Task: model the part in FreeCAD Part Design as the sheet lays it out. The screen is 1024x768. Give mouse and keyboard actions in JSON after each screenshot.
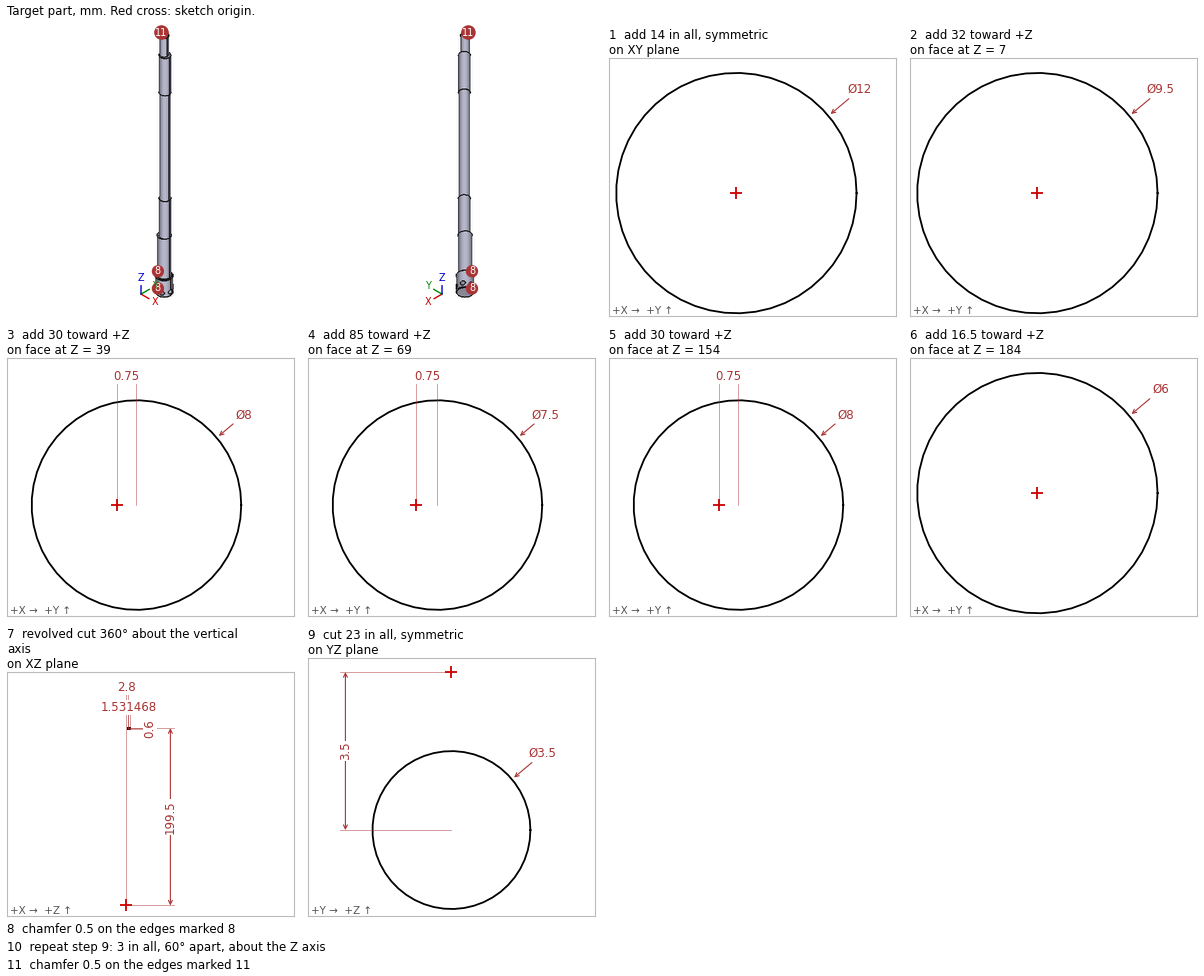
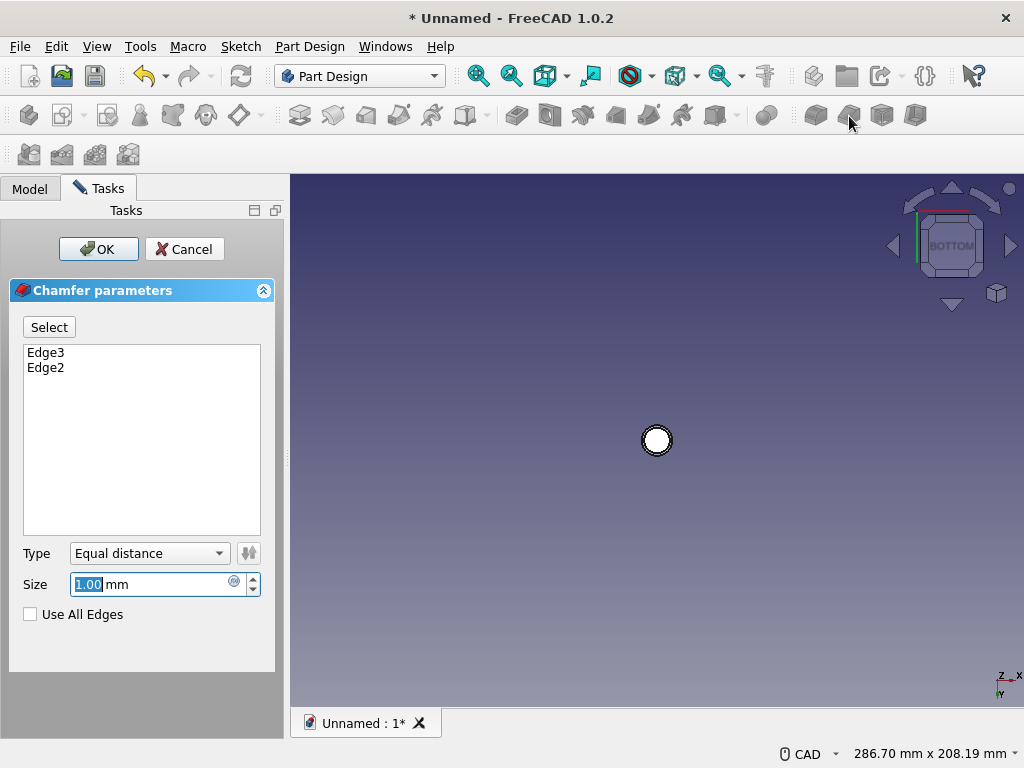
{"action": "type", "text": "0.5"}
{"action": "key", "text": "Tab"}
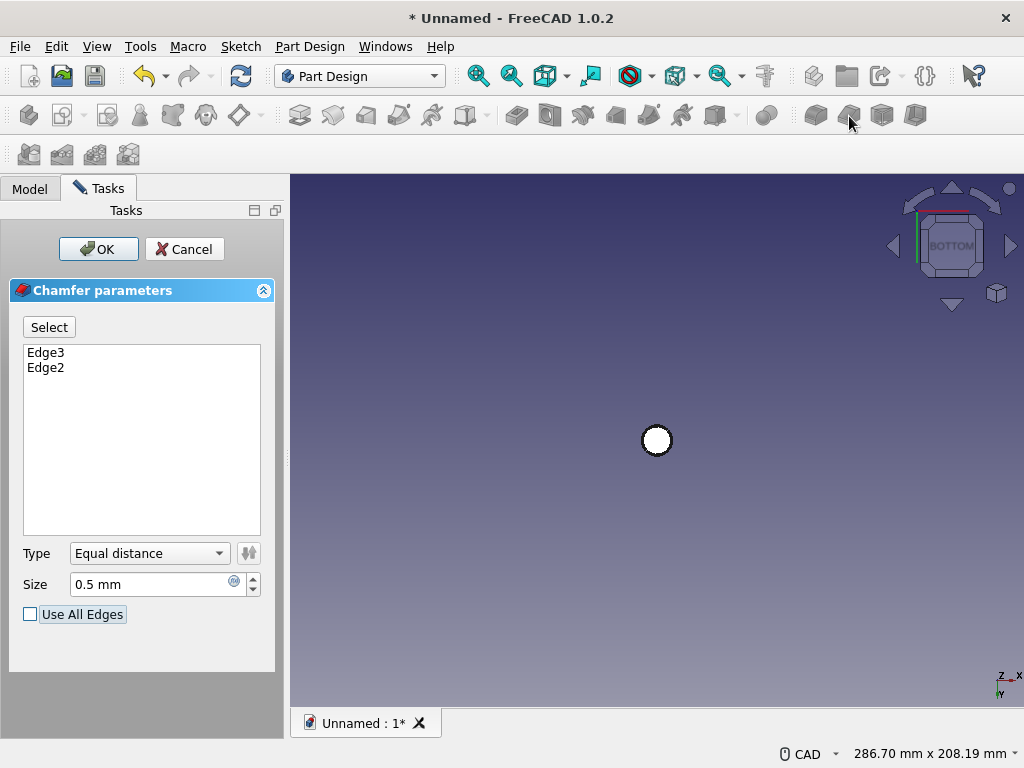
{"action": "left_click", "coordinate": [99, 249]}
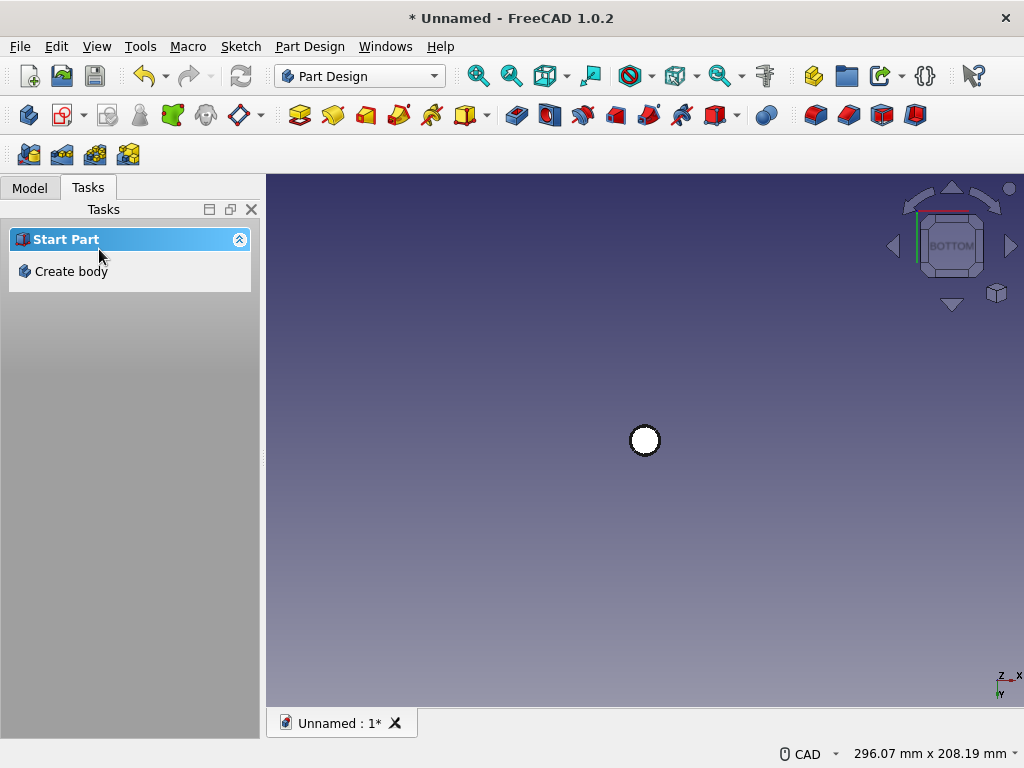
{"action": "key", "text": "v f"}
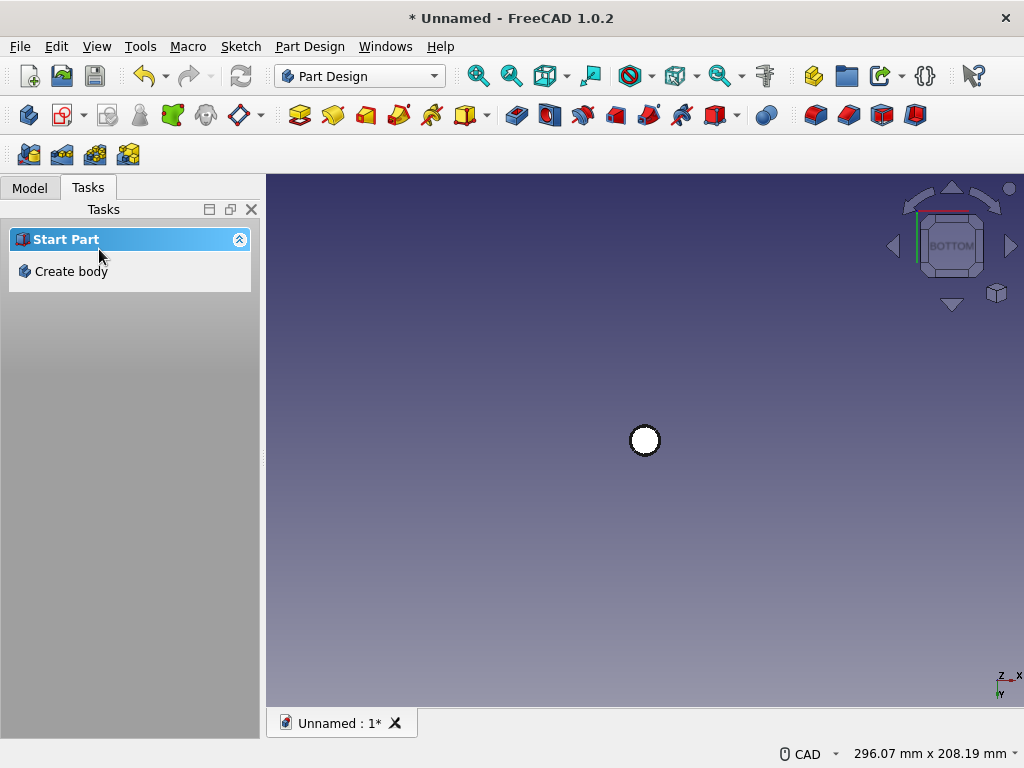
{"action": "left_click", "coordinate": [62, 116]}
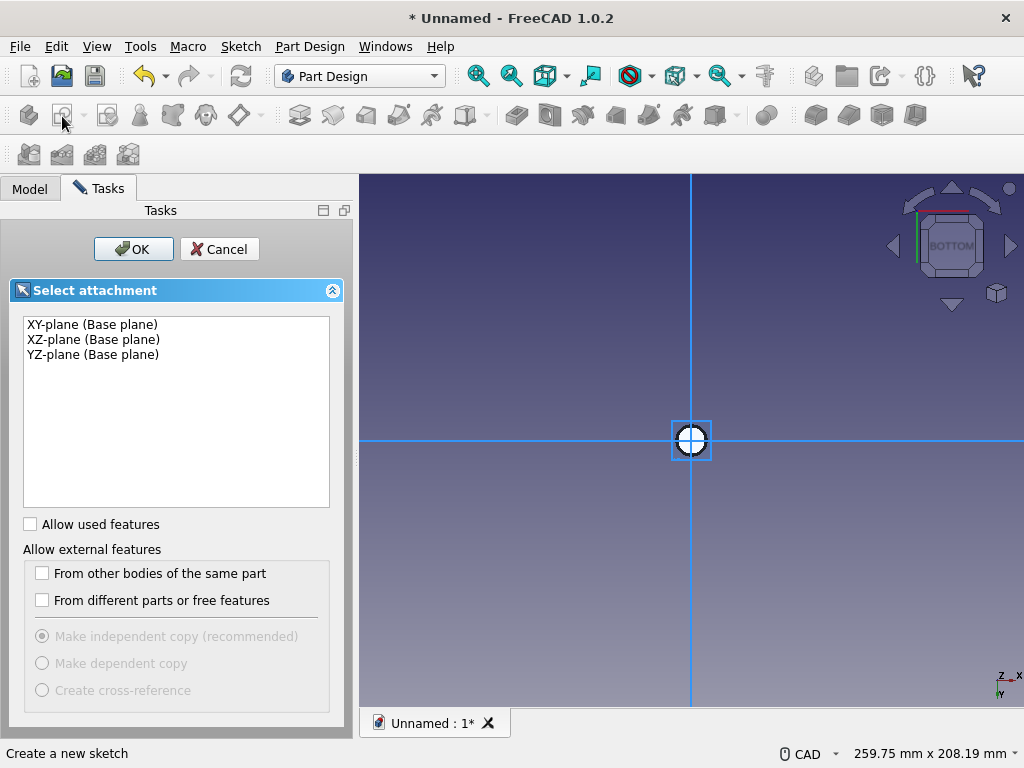
{"action": "left_click", "coordinate": [84, 354]}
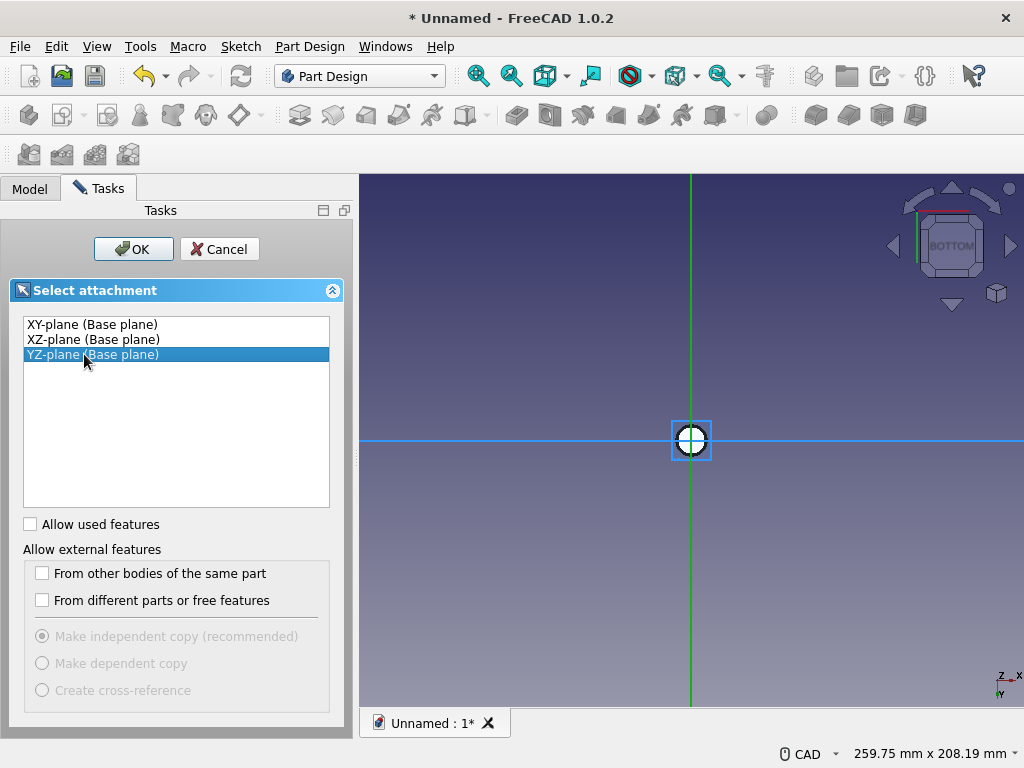
{"action": "left_click", "coordinate": [134, 249]}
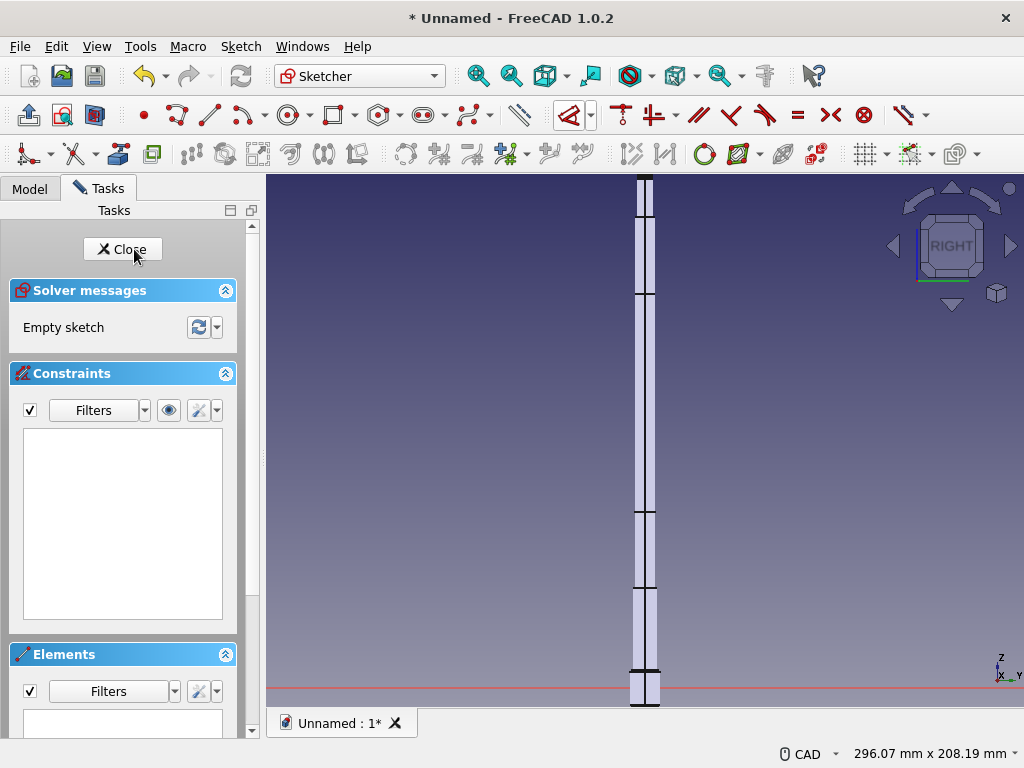
{"action": "key", "text": "q s"}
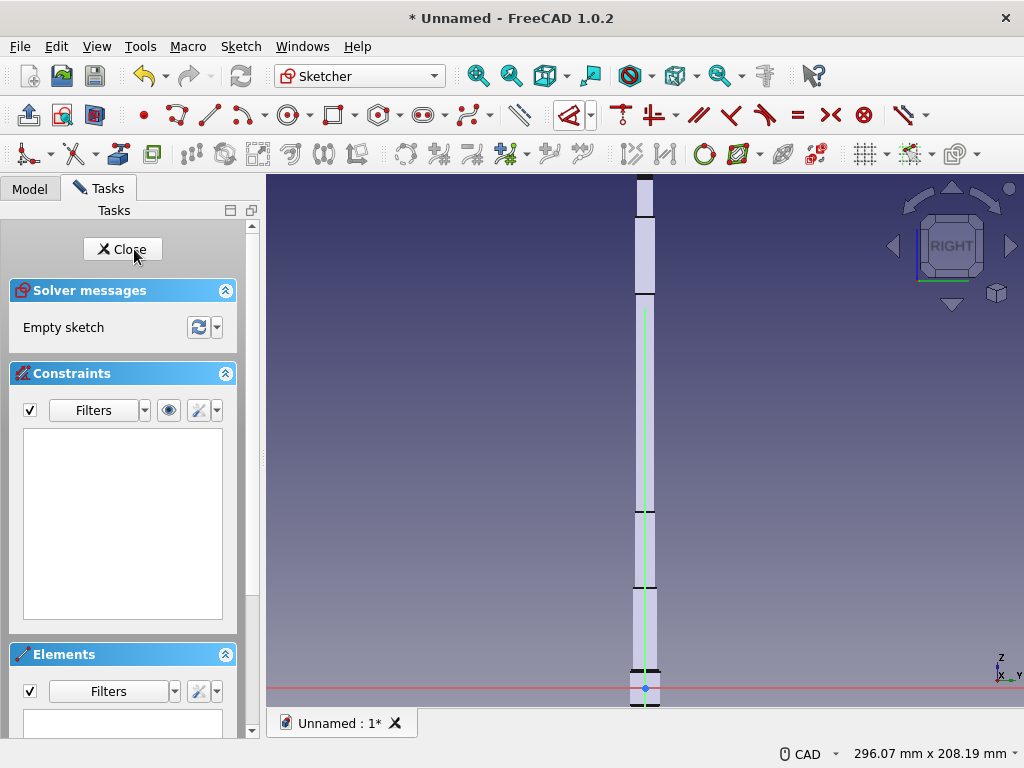
{"action": "scroll", "coordinate": [576, 440], "scroll_direction": "down", "scroll_amount": 5}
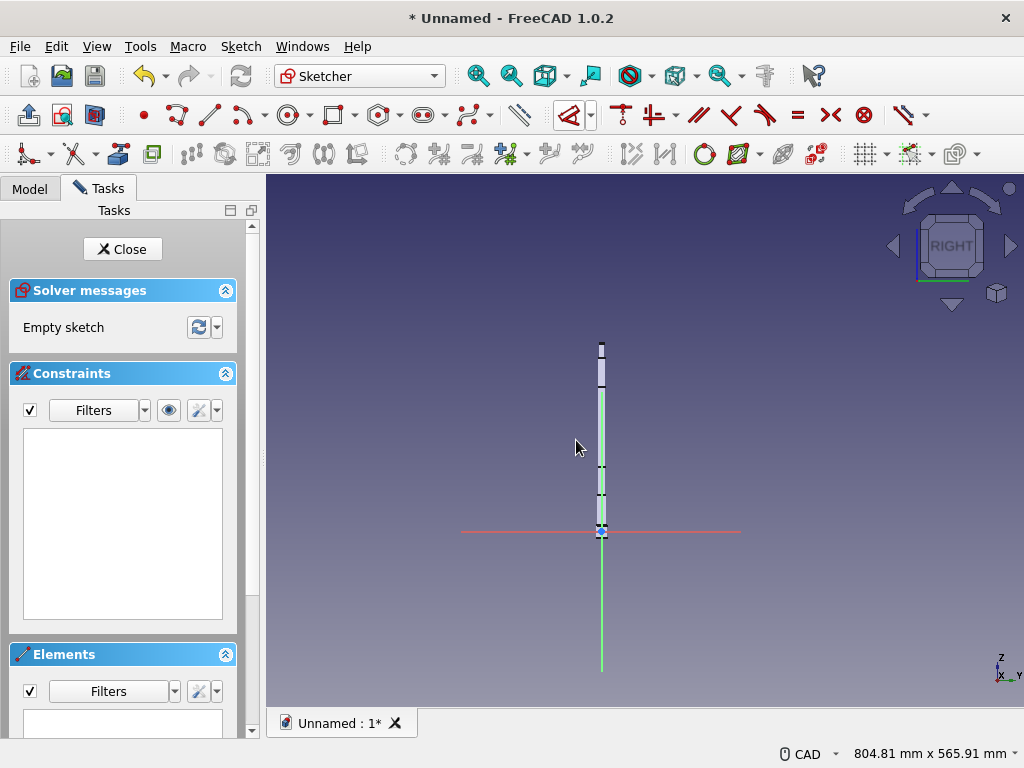
{"action": "scroll", "coordinate": [603, 539], "scroll_direction": "up", "scroll_amount": 15}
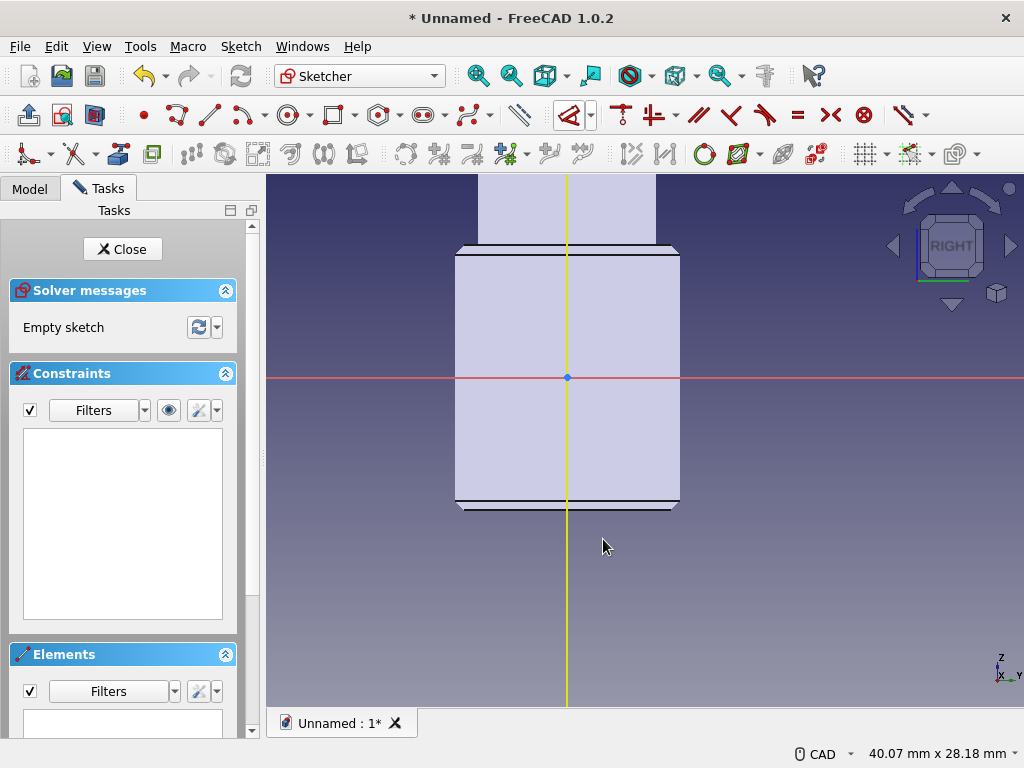
{"action": "scroll", "coordinate": [563, 422], "scroll_direction": "up", "scroll_amount": 6}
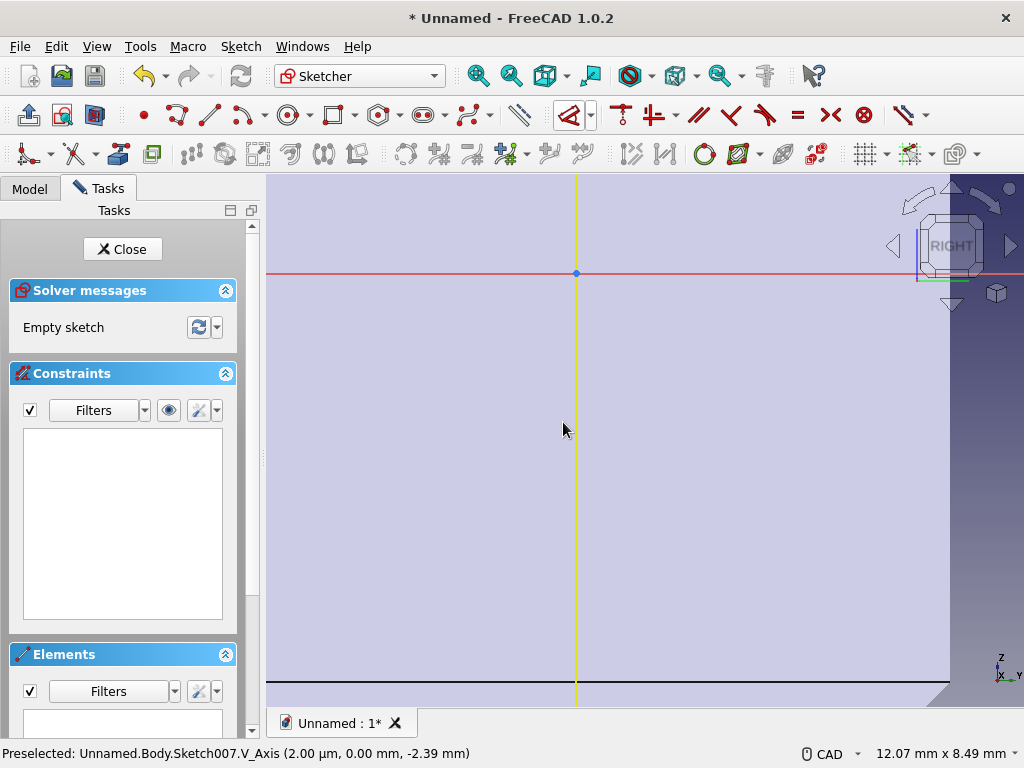
{"action": "key", "text": "g c"}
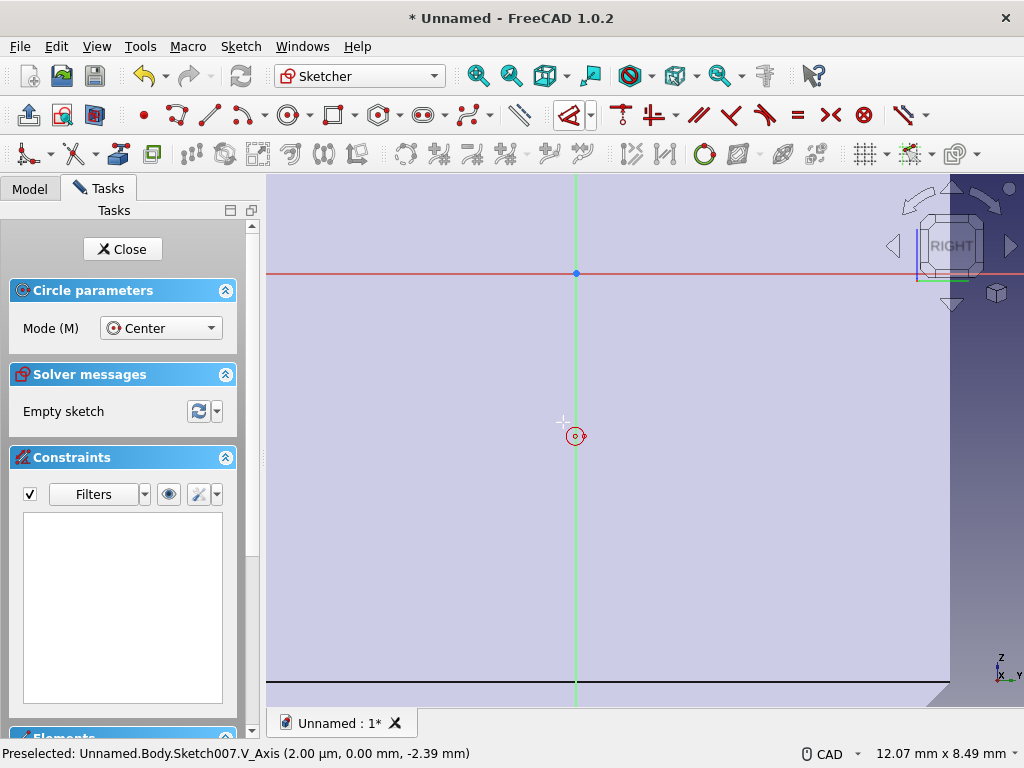
{"action": "left_click", "coordinate": [576, 494]}
{"action": "left_click", "coordinate": [654, 416]}
{"action": "key", "text": "Escape"}